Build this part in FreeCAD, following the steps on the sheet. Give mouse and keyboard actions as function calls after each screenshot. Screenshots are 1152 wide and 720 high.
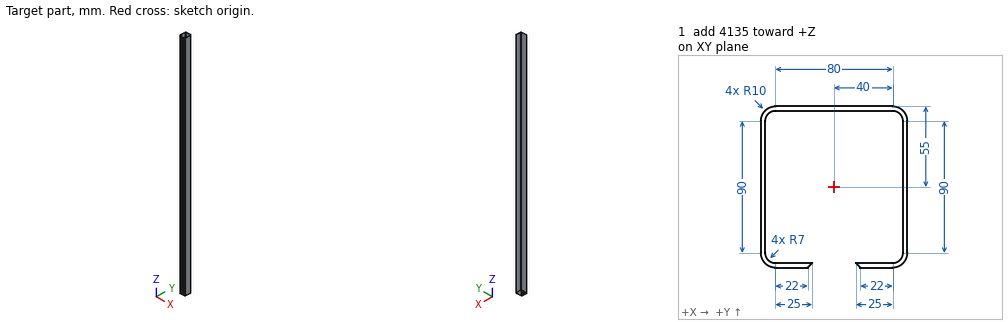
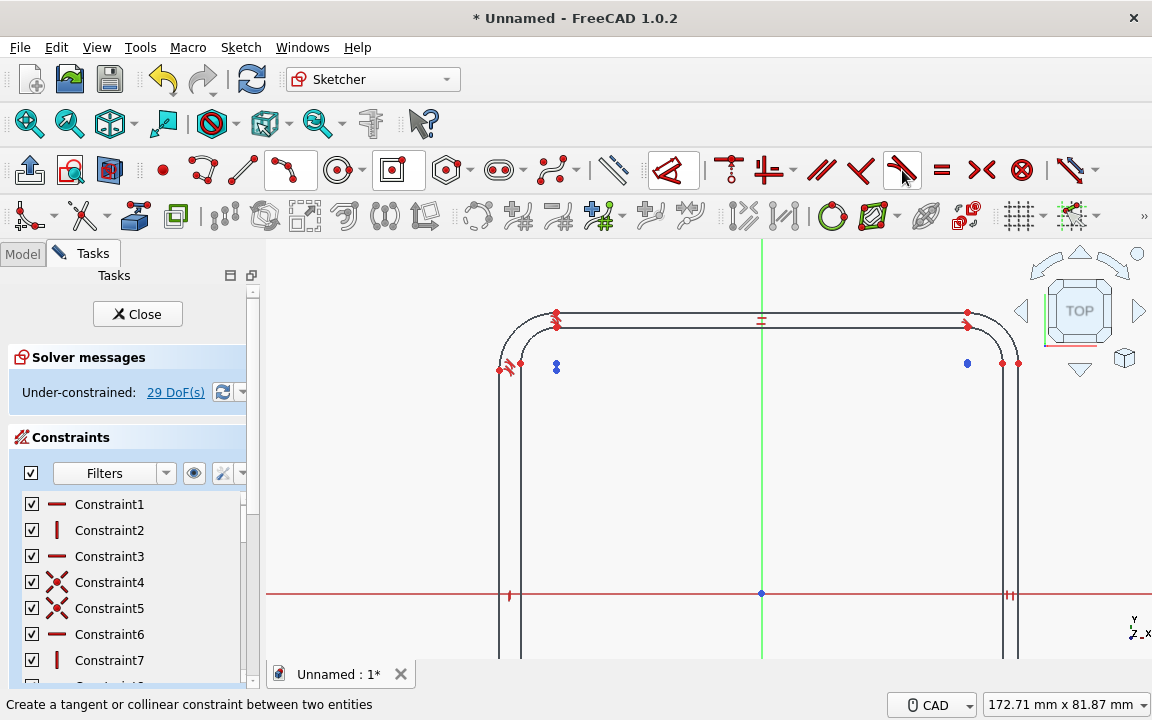
click(680, 328)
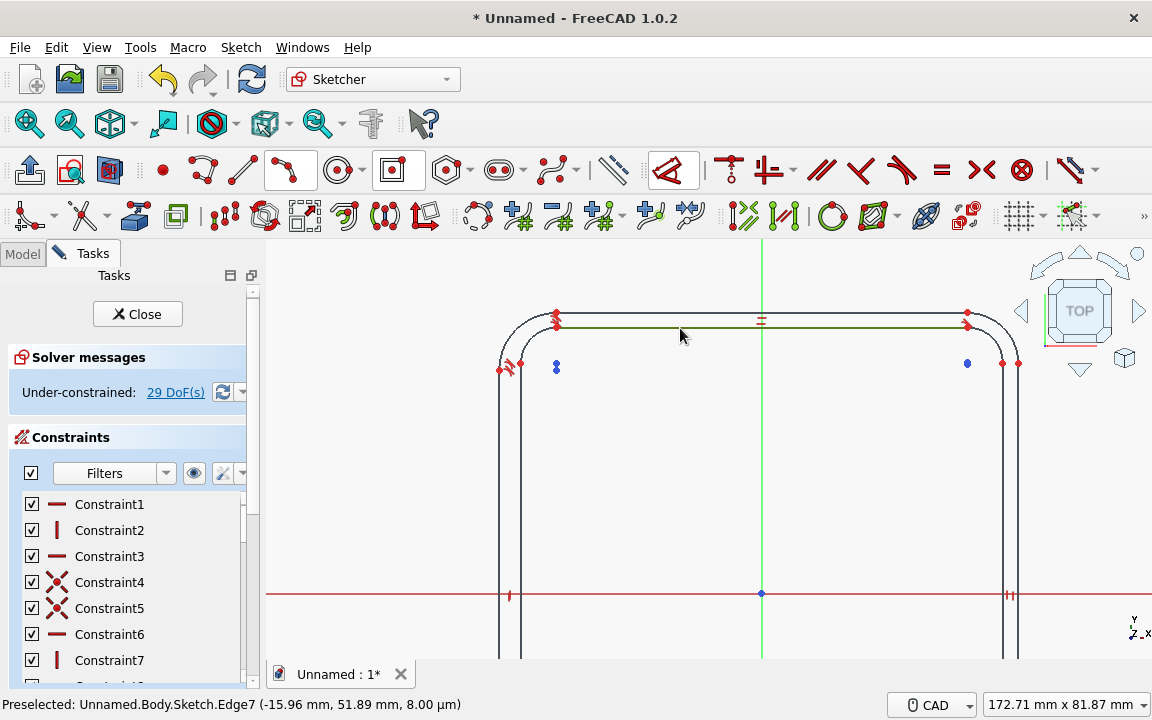
click(984, 331)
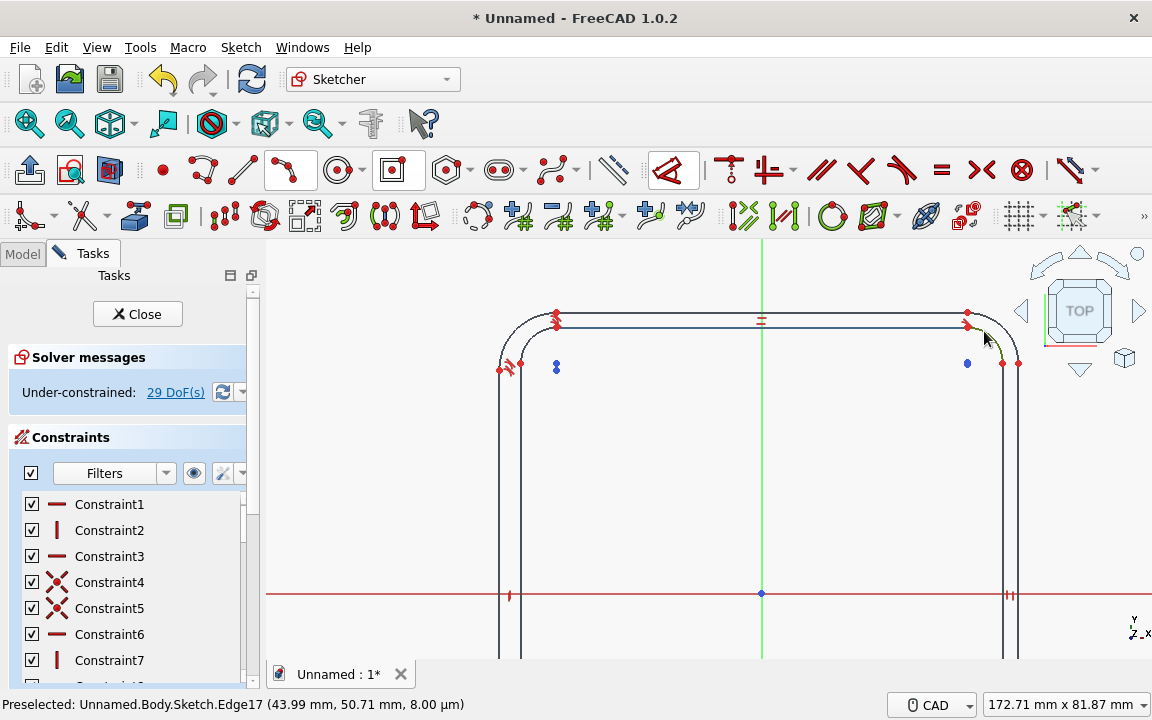
click(902, 170)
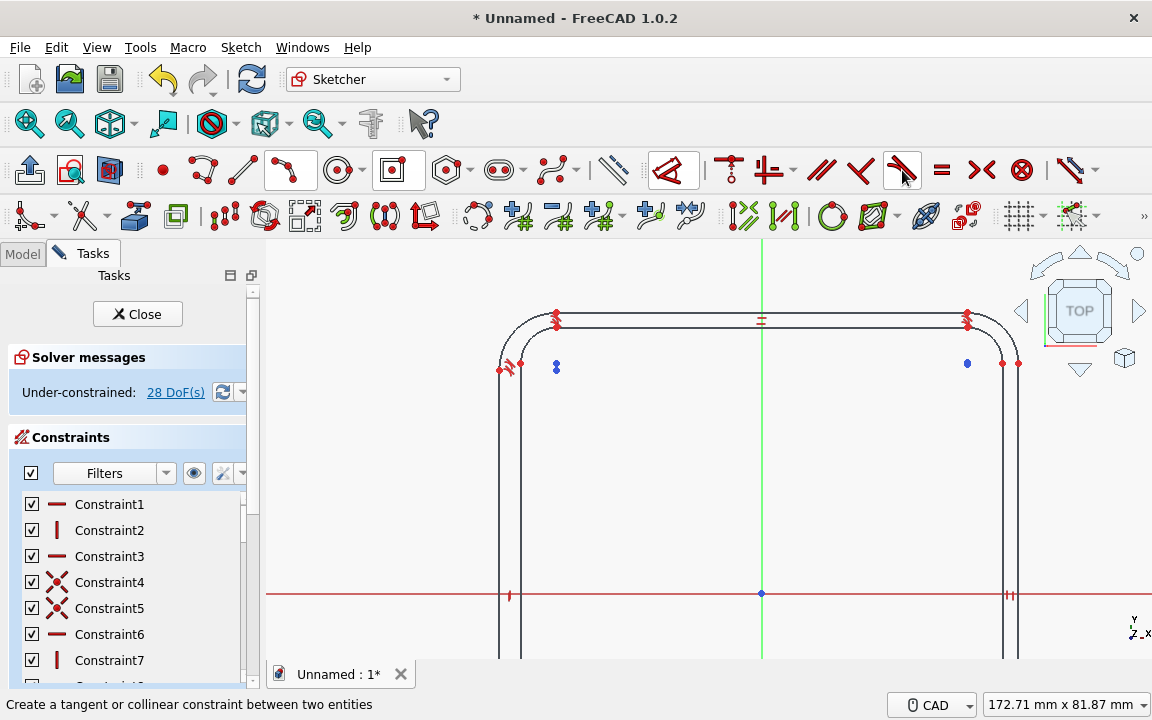
scroll(541, 331, down, 4)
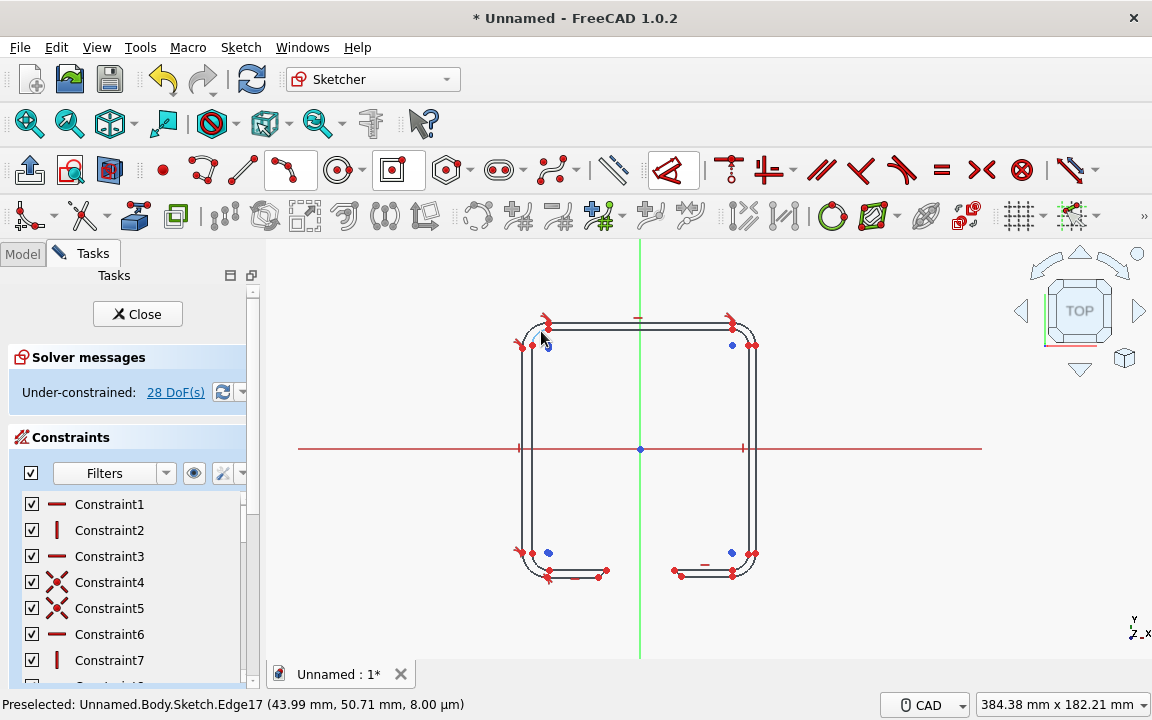
scroll(749, 408, up, 4)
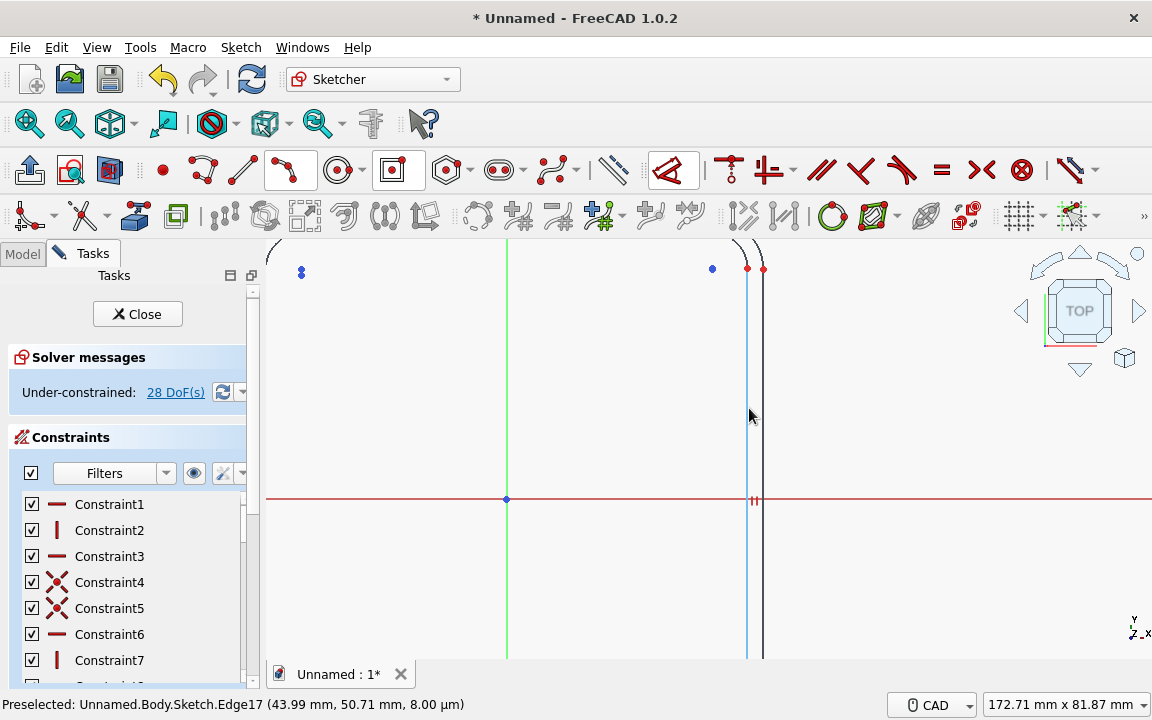
click(747, 408)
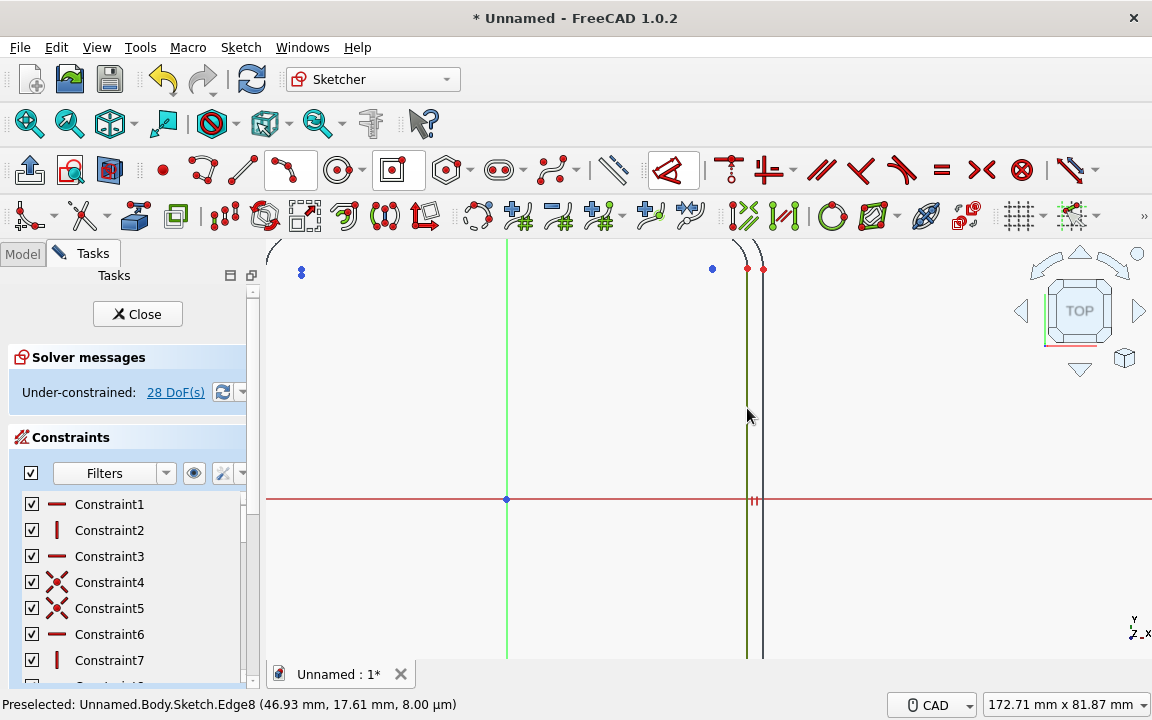
scroll(750, 408, down, 4)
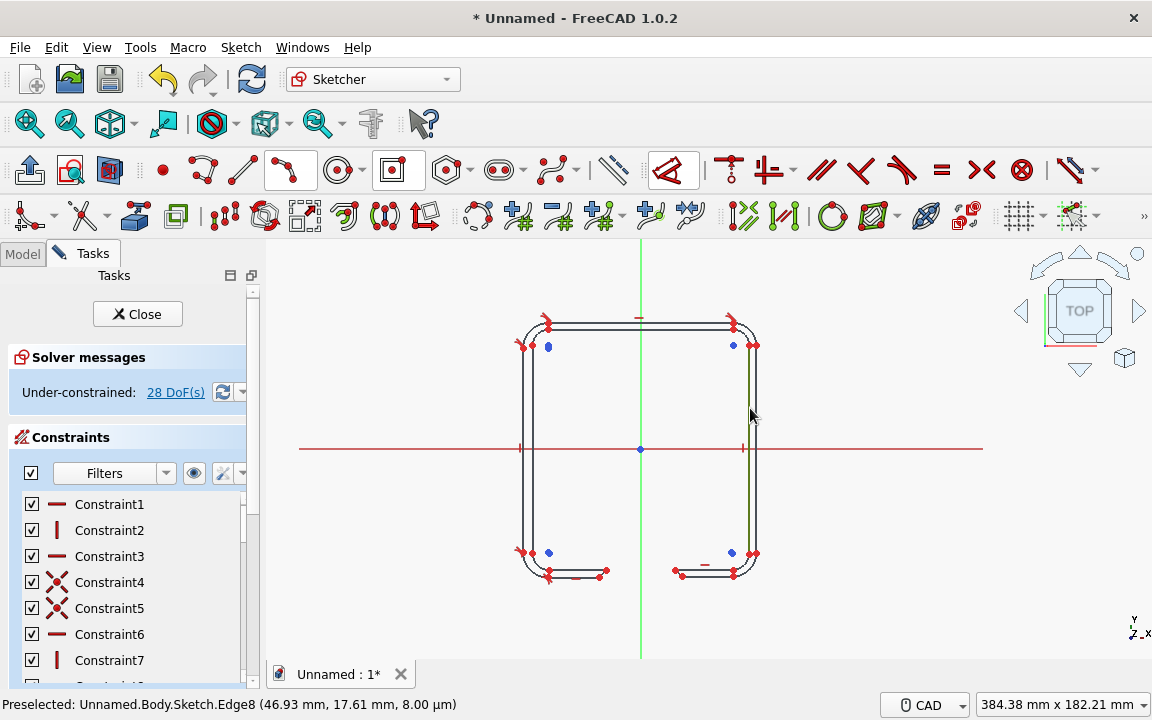
scroll(748, 338, up, 4)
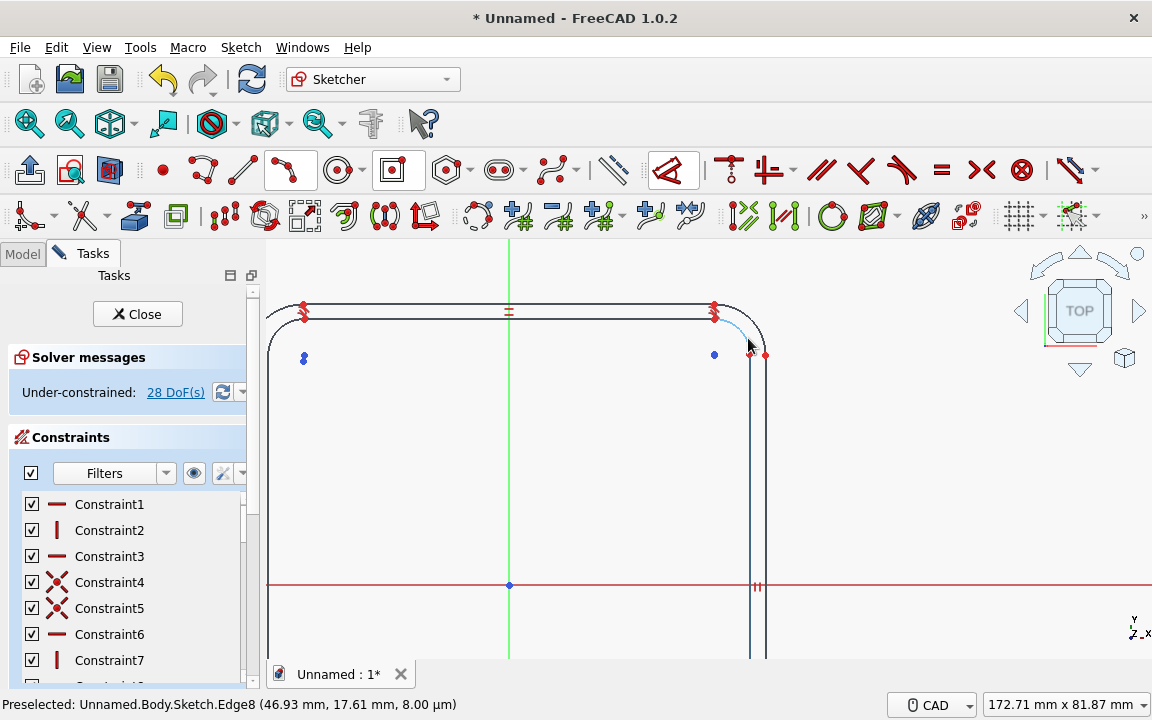
click(746, 339)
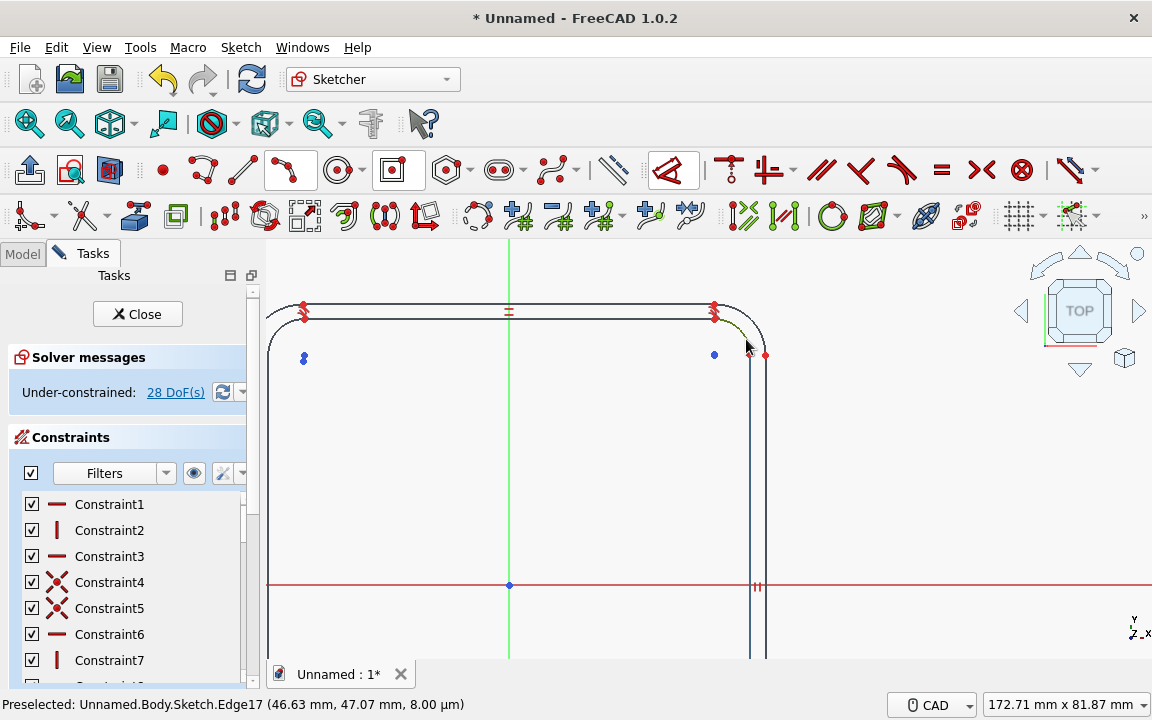
click(902, 170)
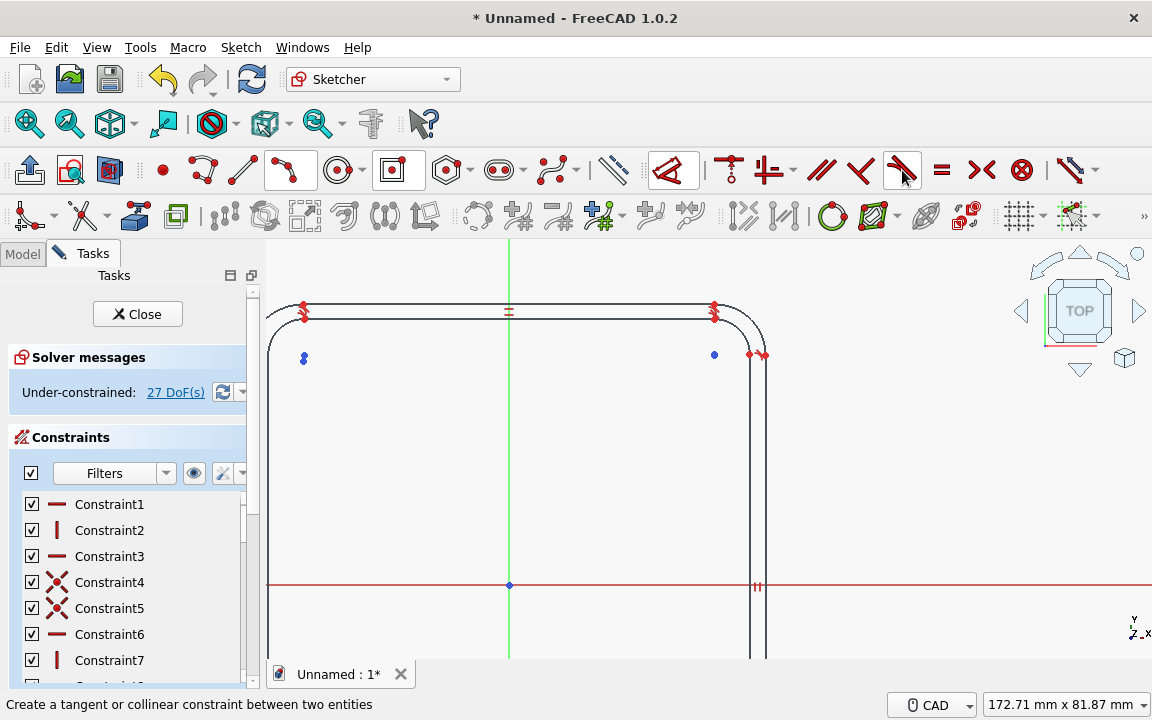
click(750, 494)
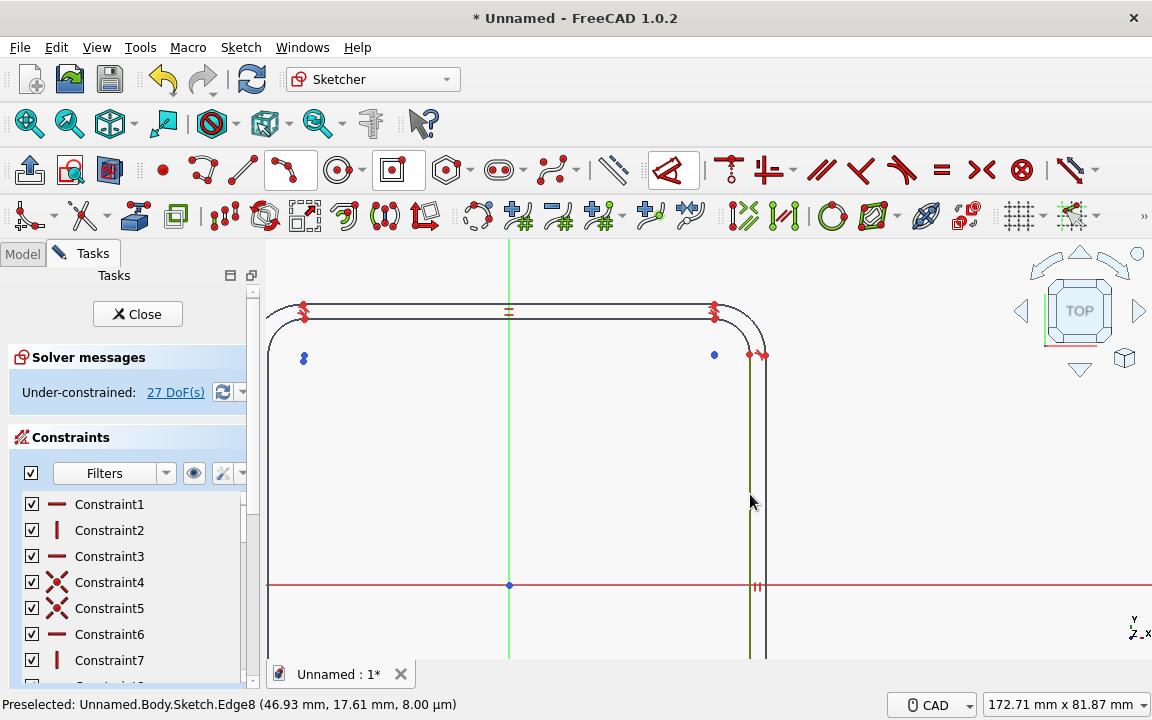
scroll(748, 338, down, 4)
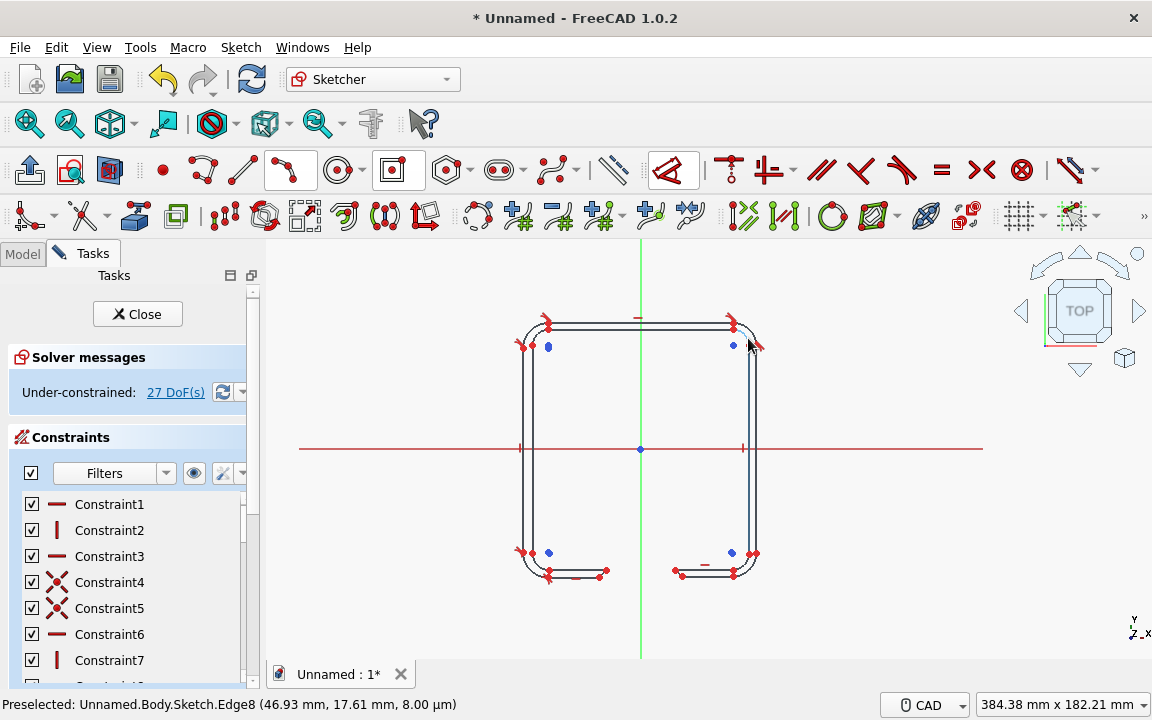
scroll(740, 568, up, 4)